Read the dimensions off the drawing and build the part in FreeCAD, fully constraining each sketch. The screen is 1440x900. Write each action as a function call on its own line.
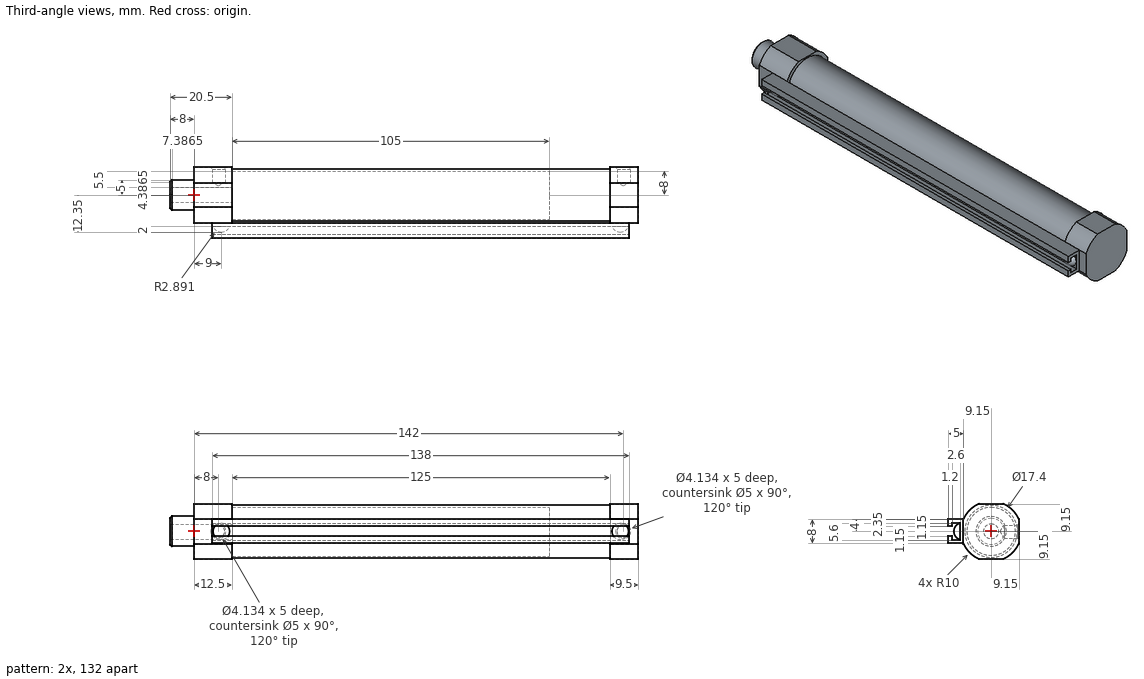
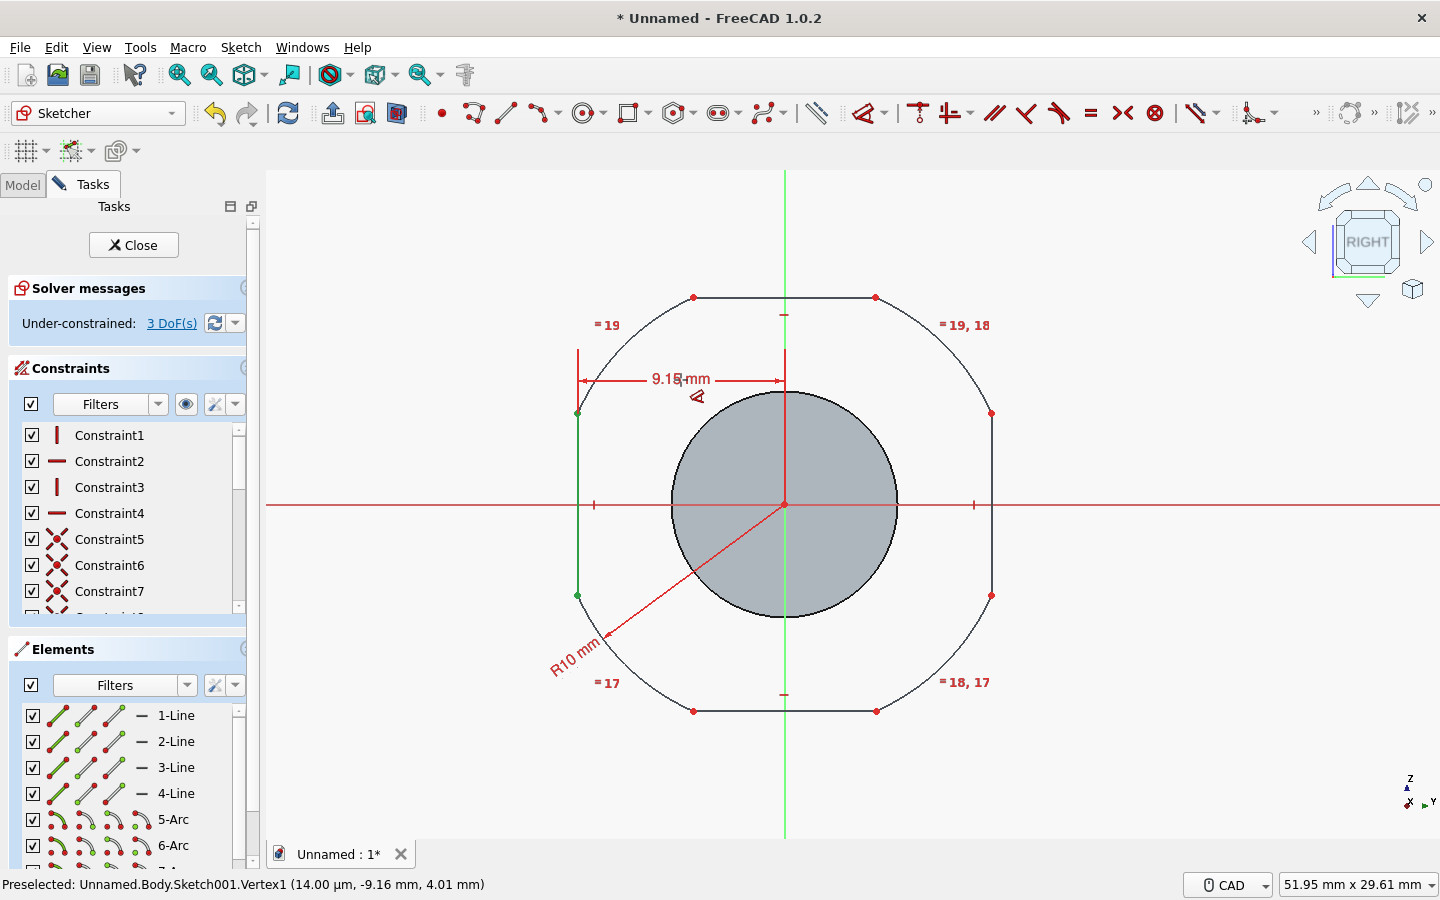
click(693, 711)
click(659, 608)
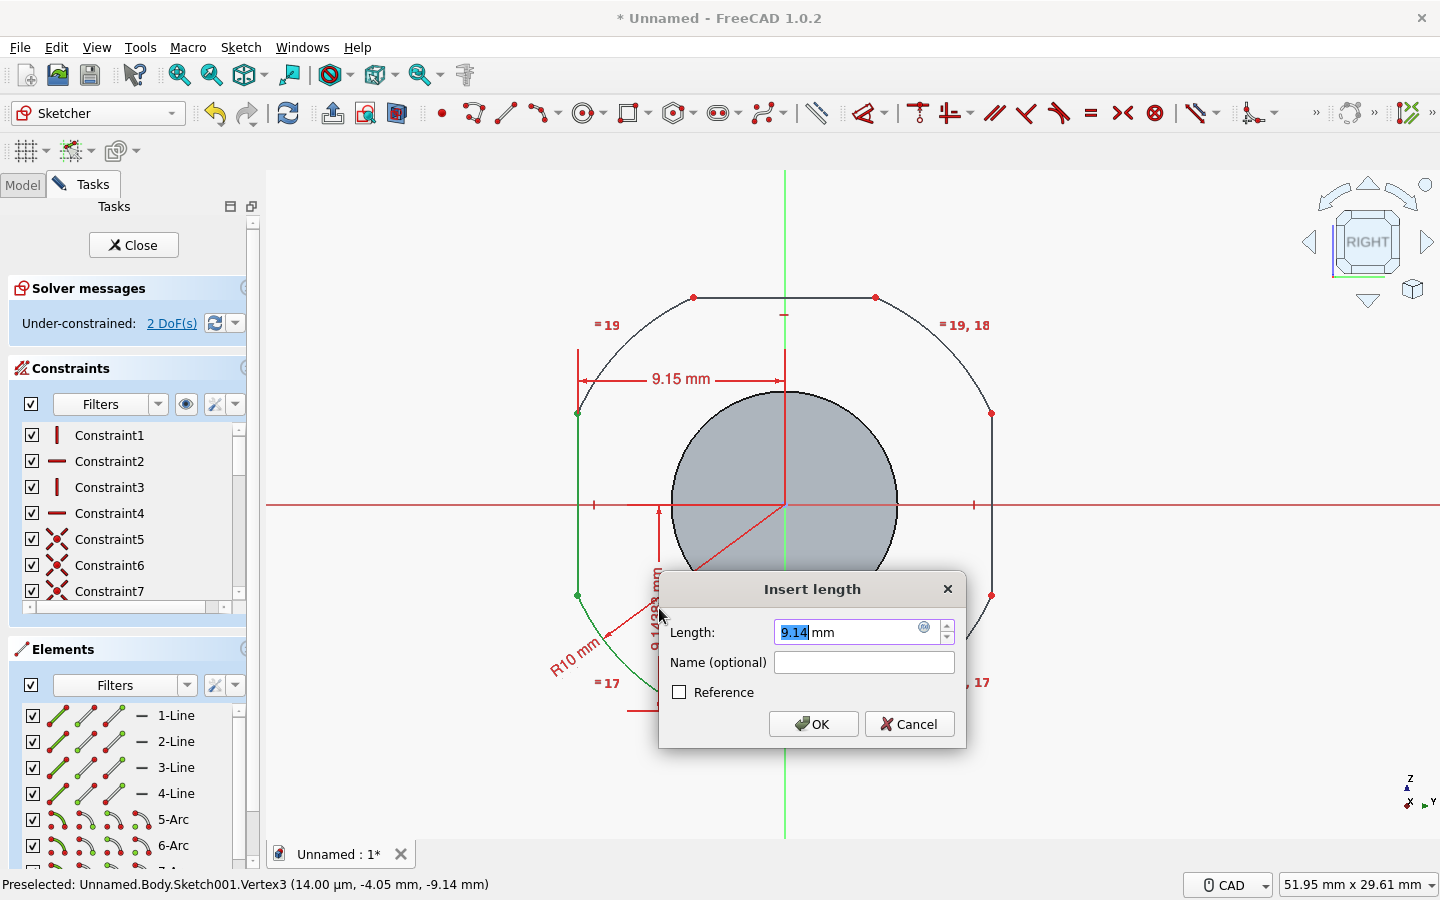
text(9.15)
key(Return)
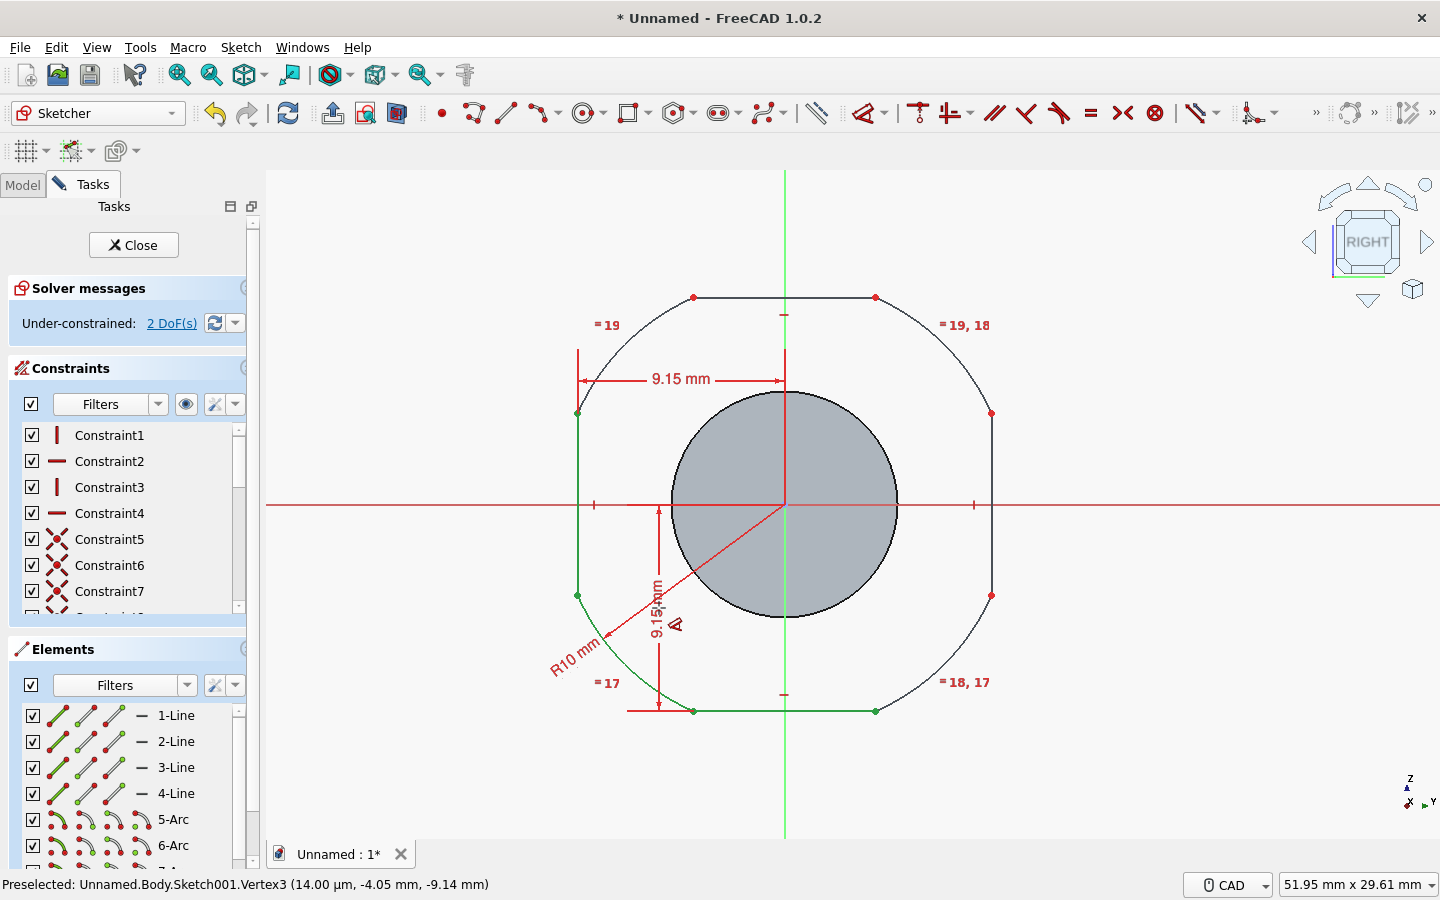
click(992, 595)
click(888, 629)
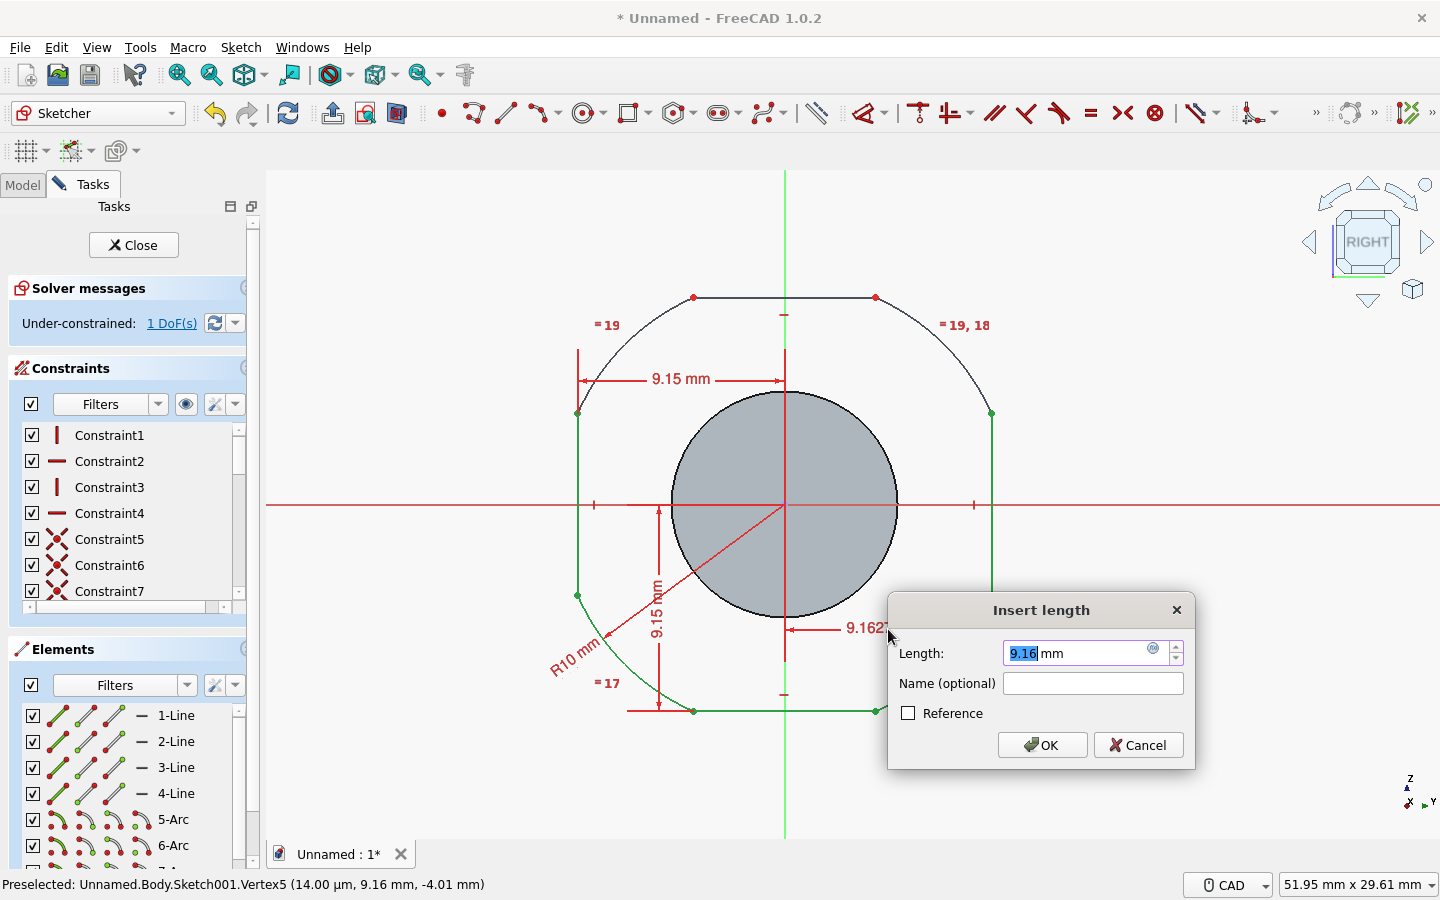
text(9.15)
key(Return)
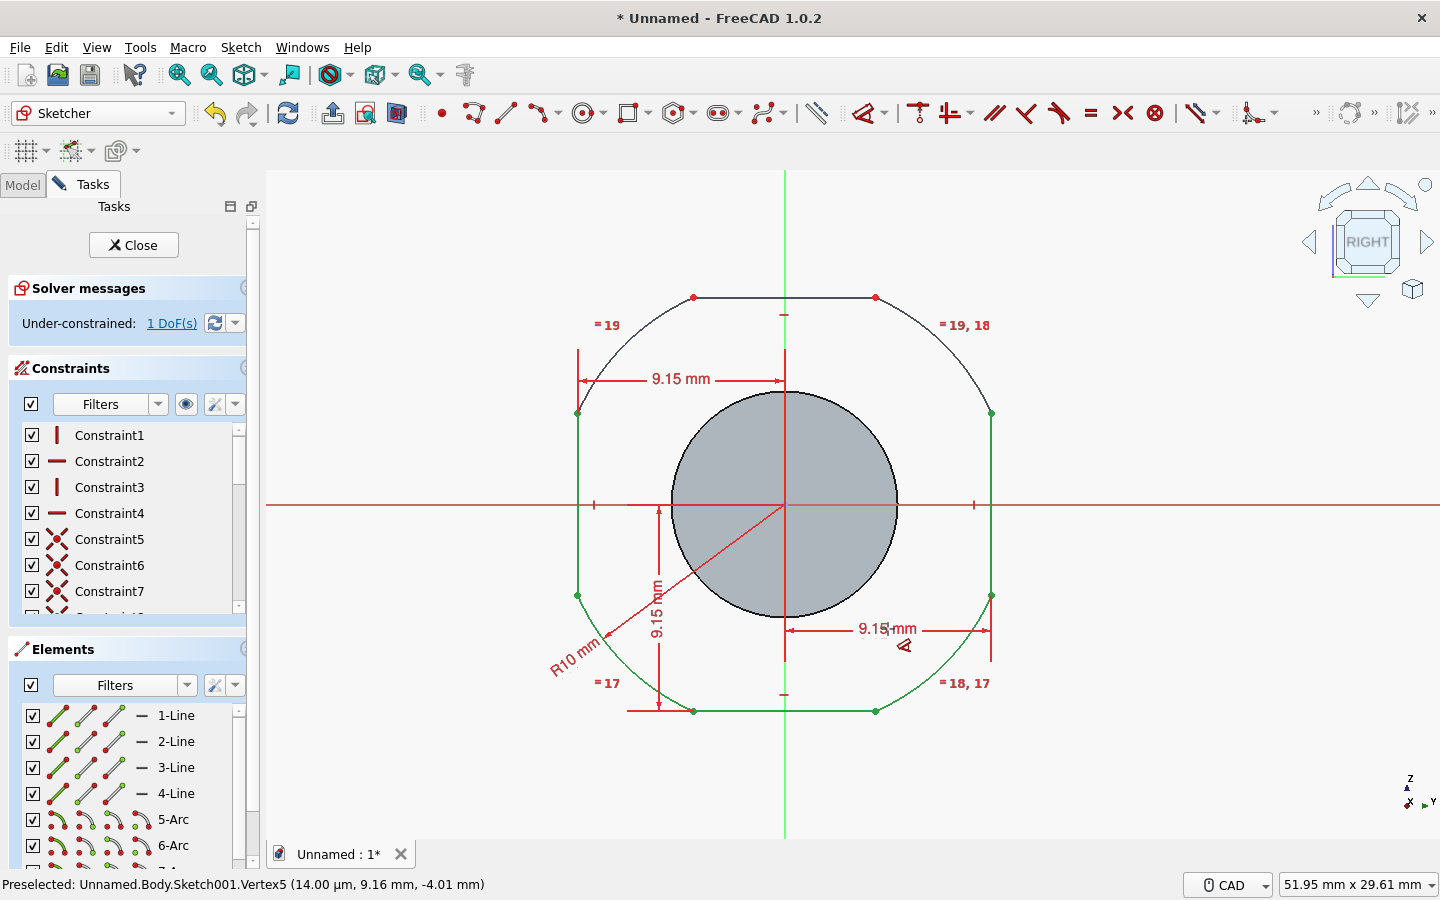
click(876, 298)
click(910, 401)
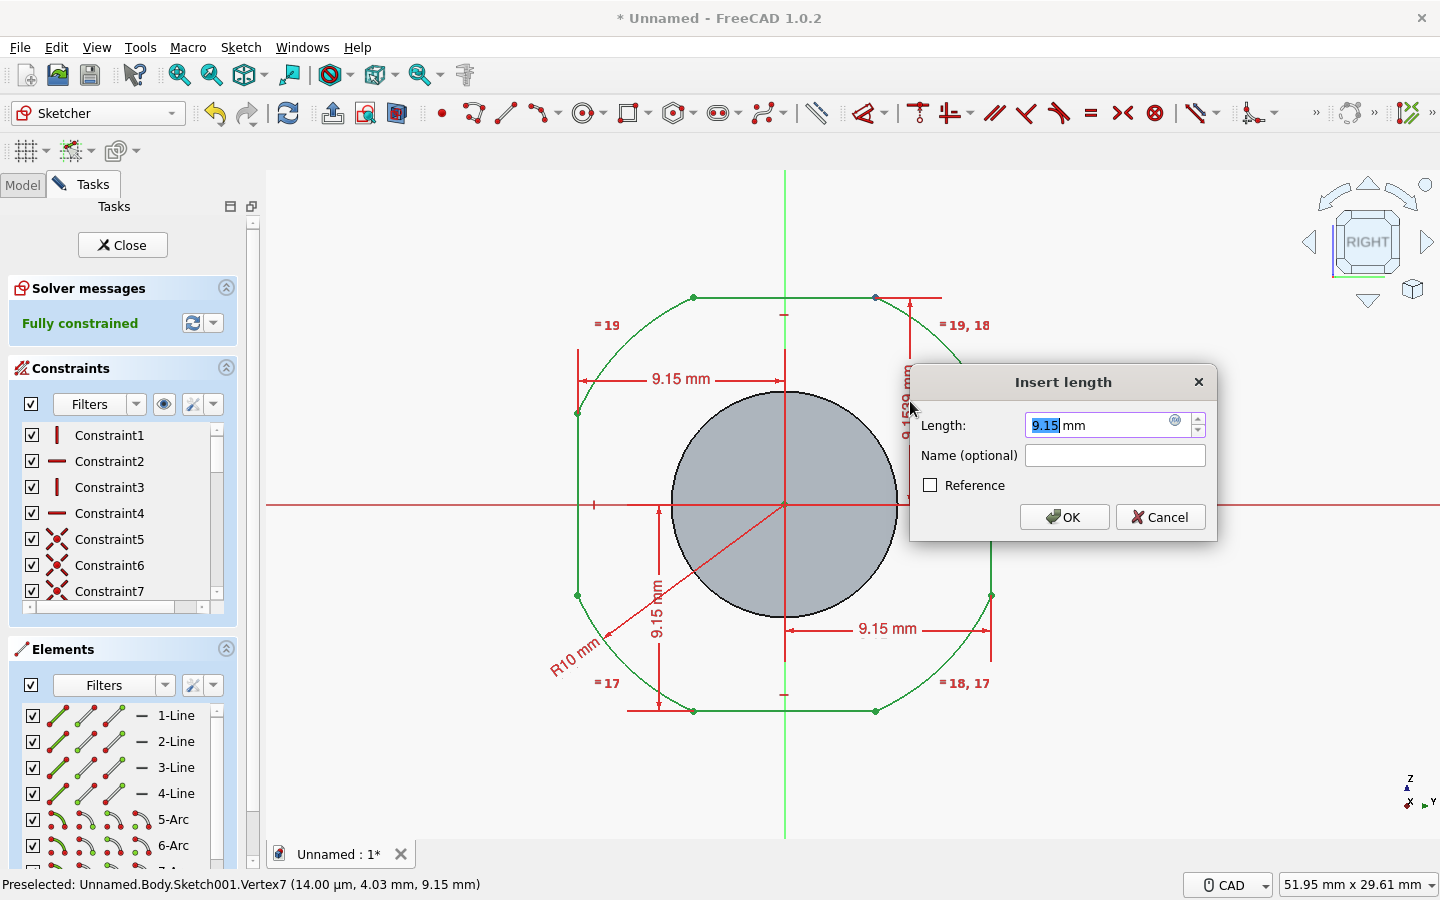
text(9.15)
key(Return)
key(Escape)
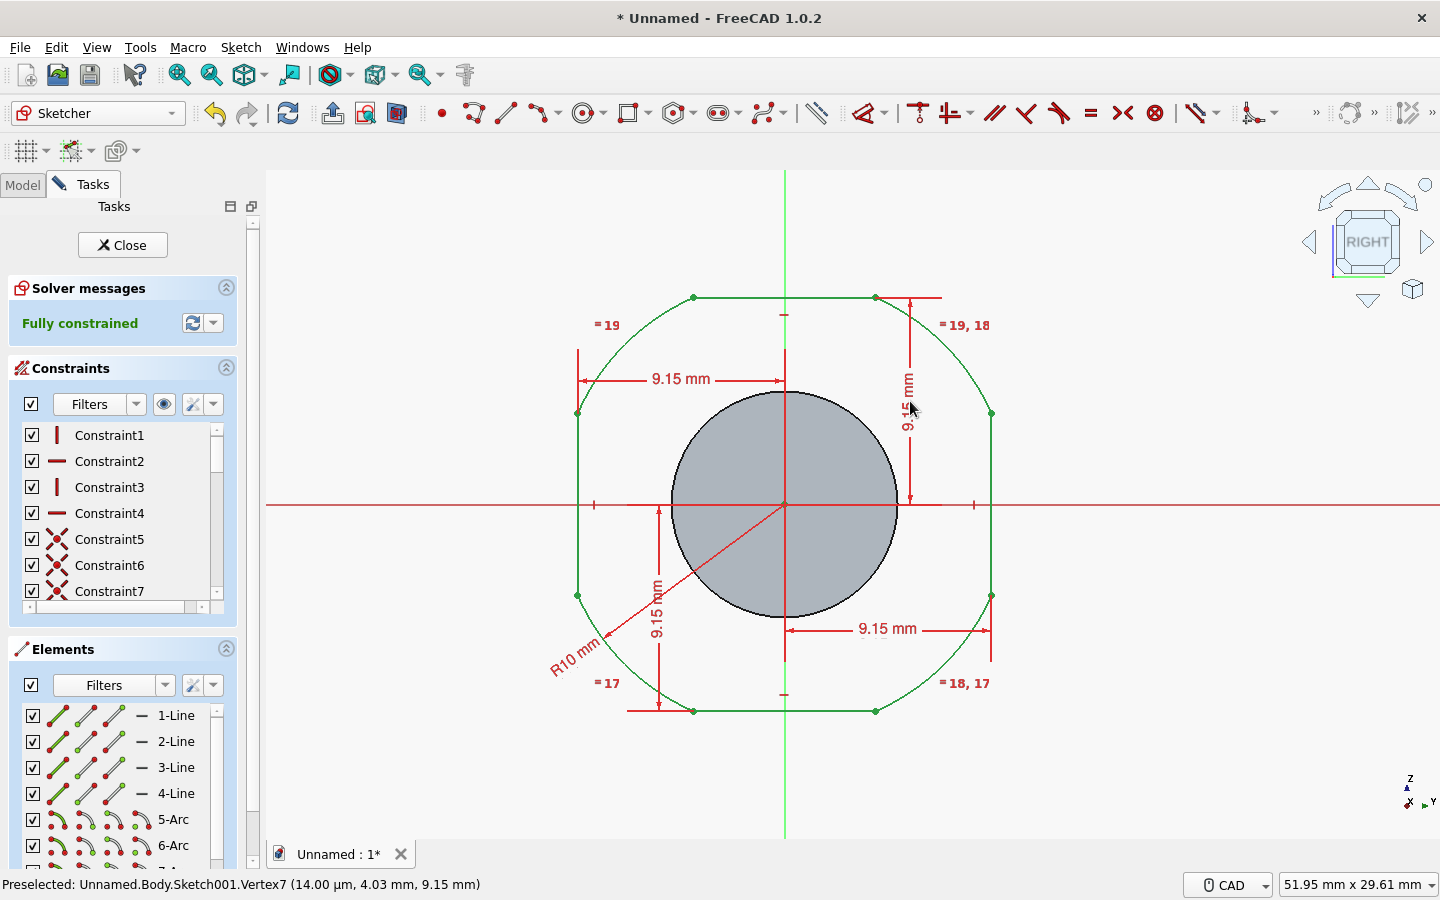
click(123, 245)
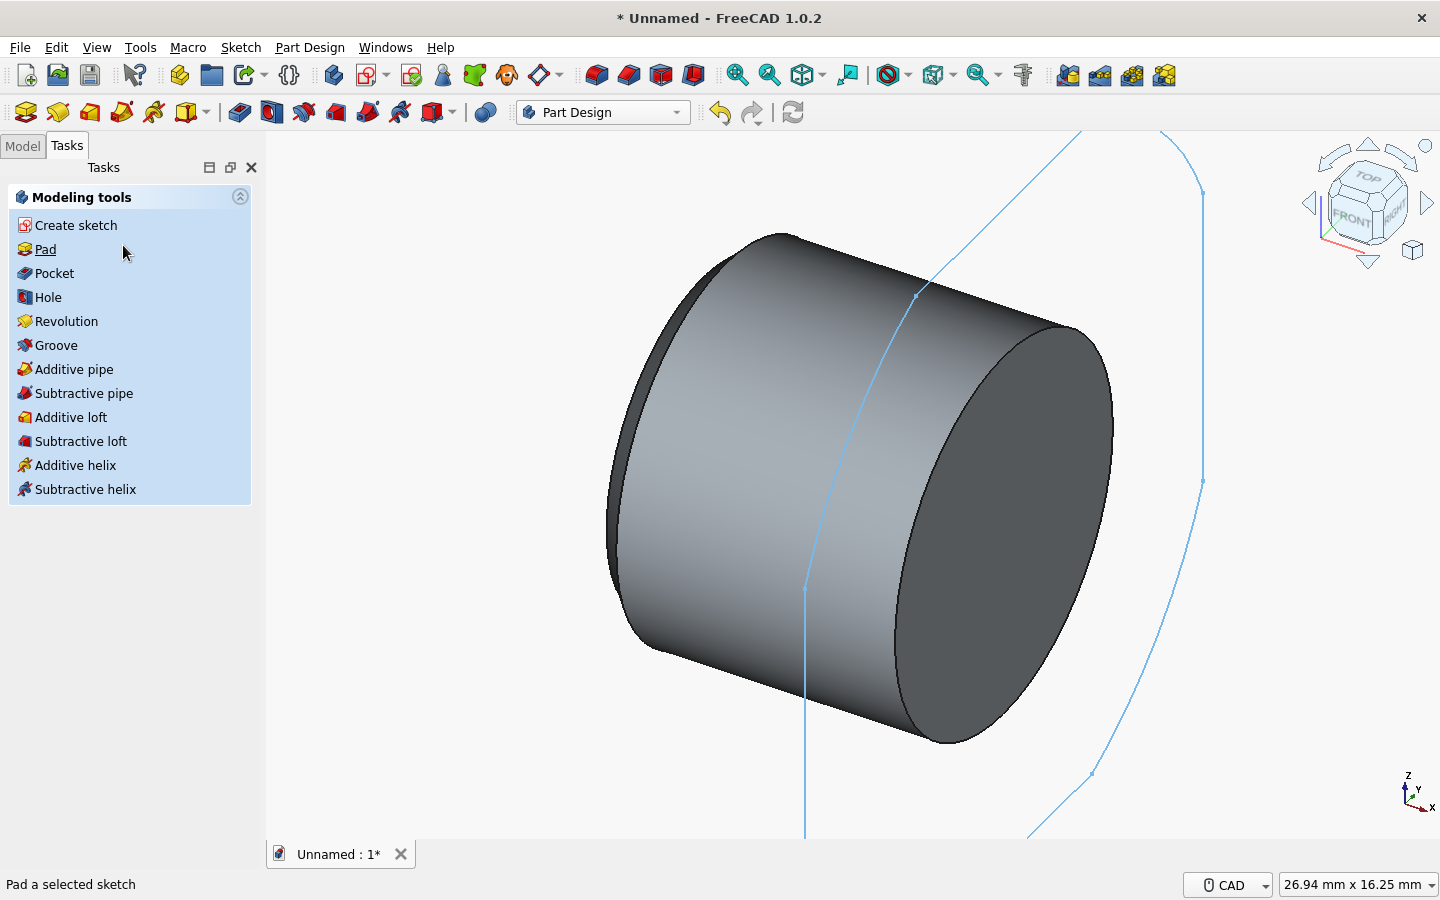
click(26, 112)